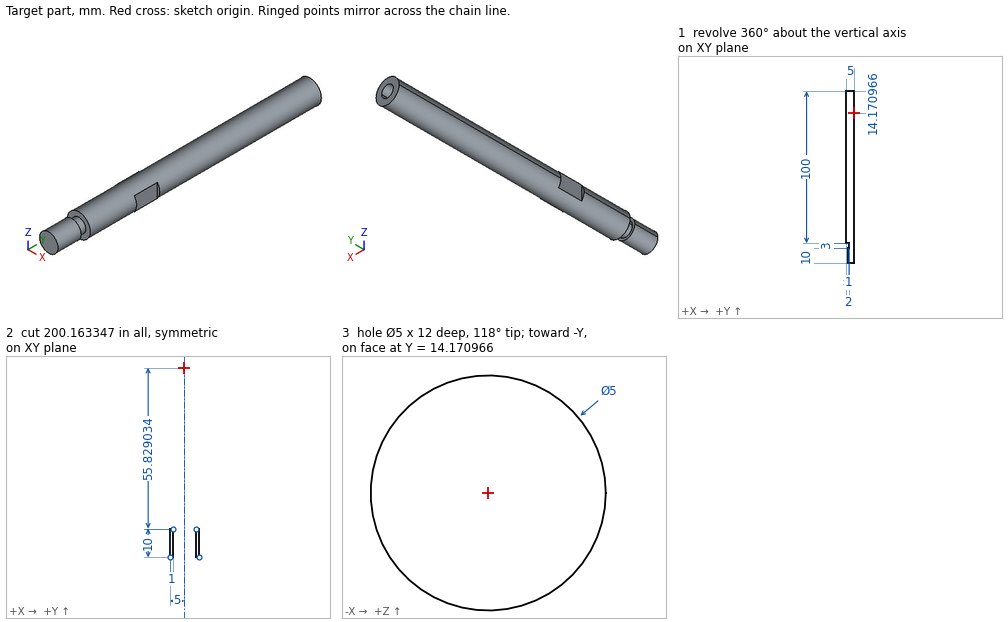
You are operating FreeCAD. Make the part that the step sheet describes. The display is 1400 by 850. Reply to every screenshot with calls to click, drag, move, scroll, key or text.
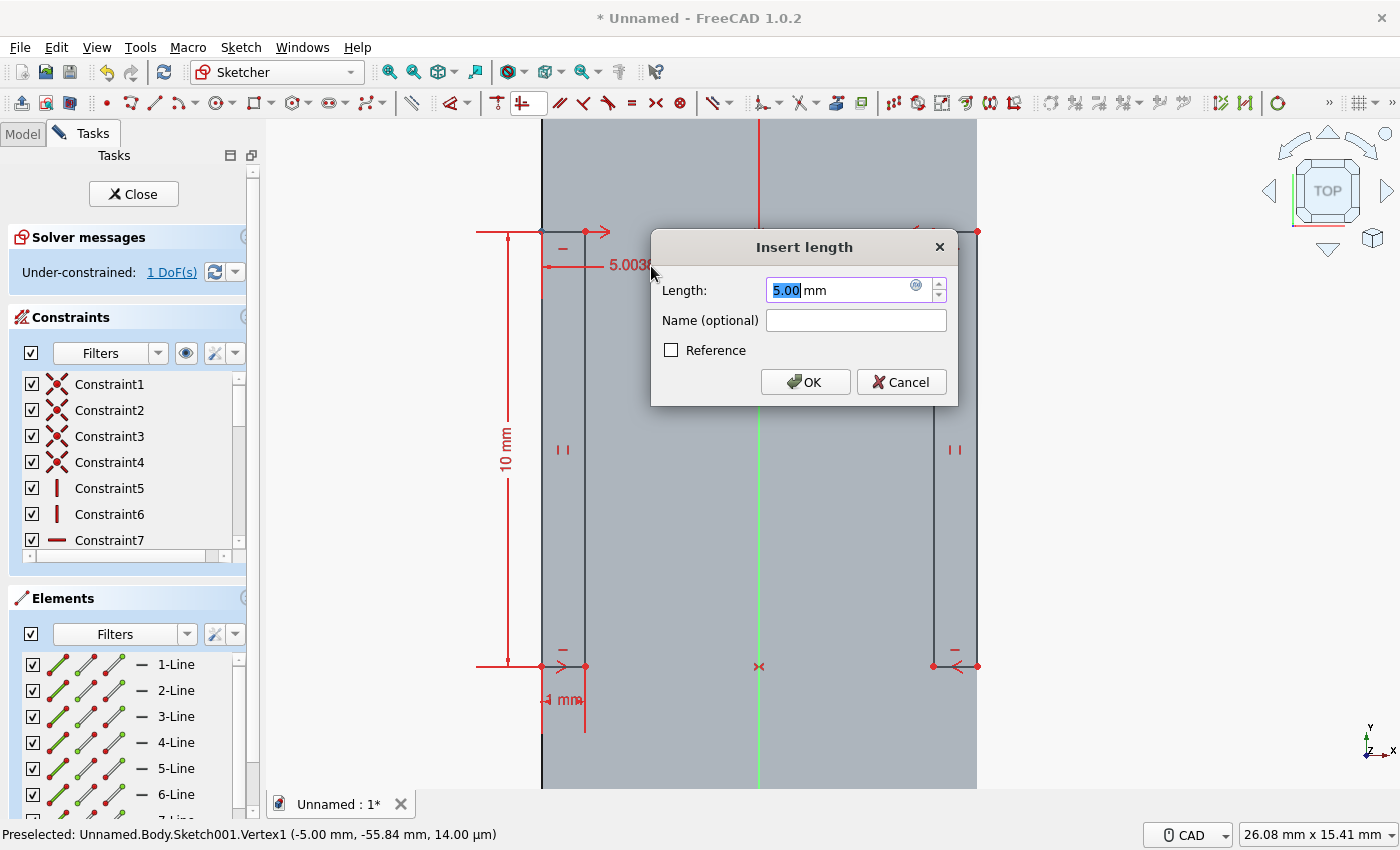
text(5)
key(Return)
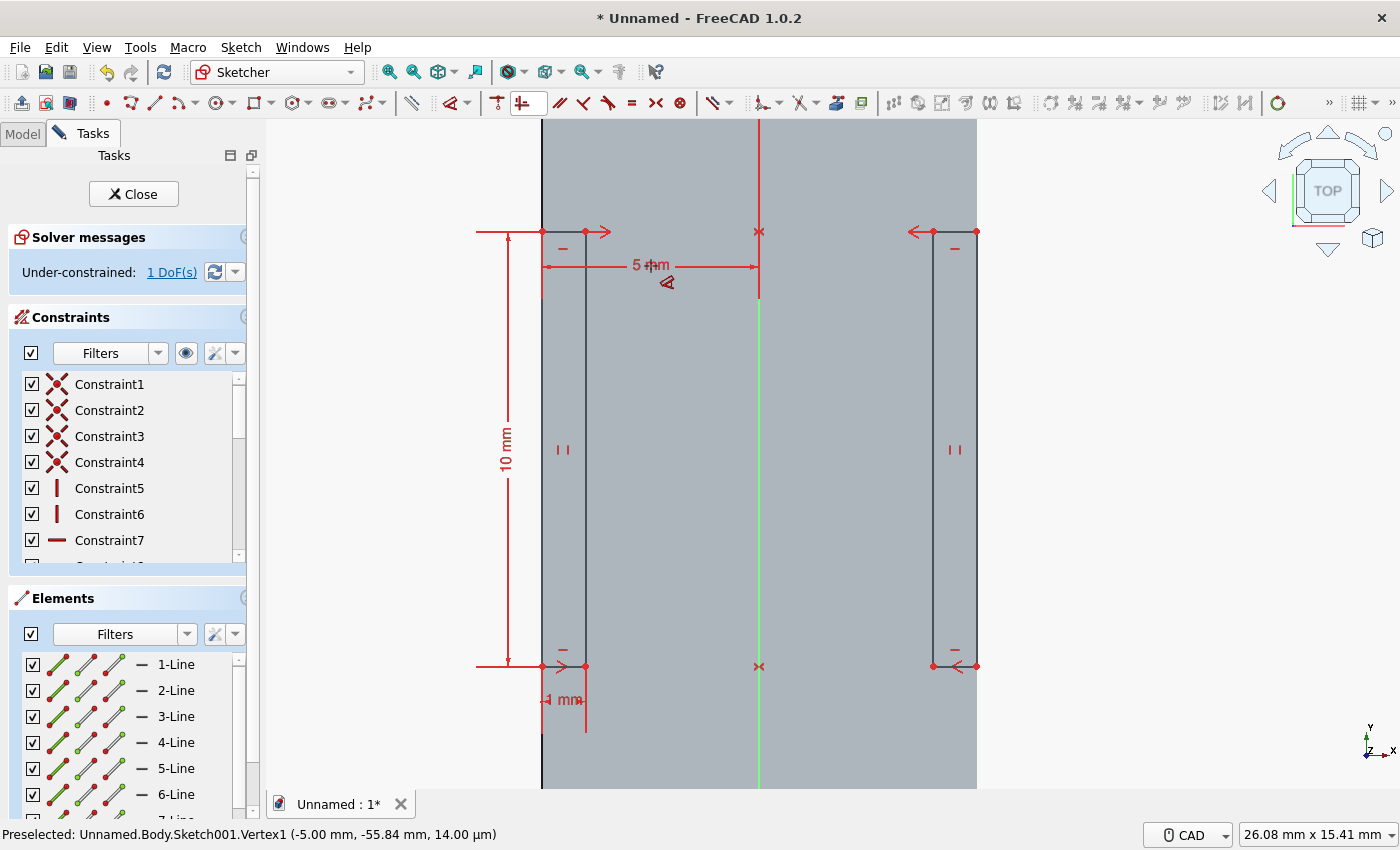
click(542, 232)
click(508, 189)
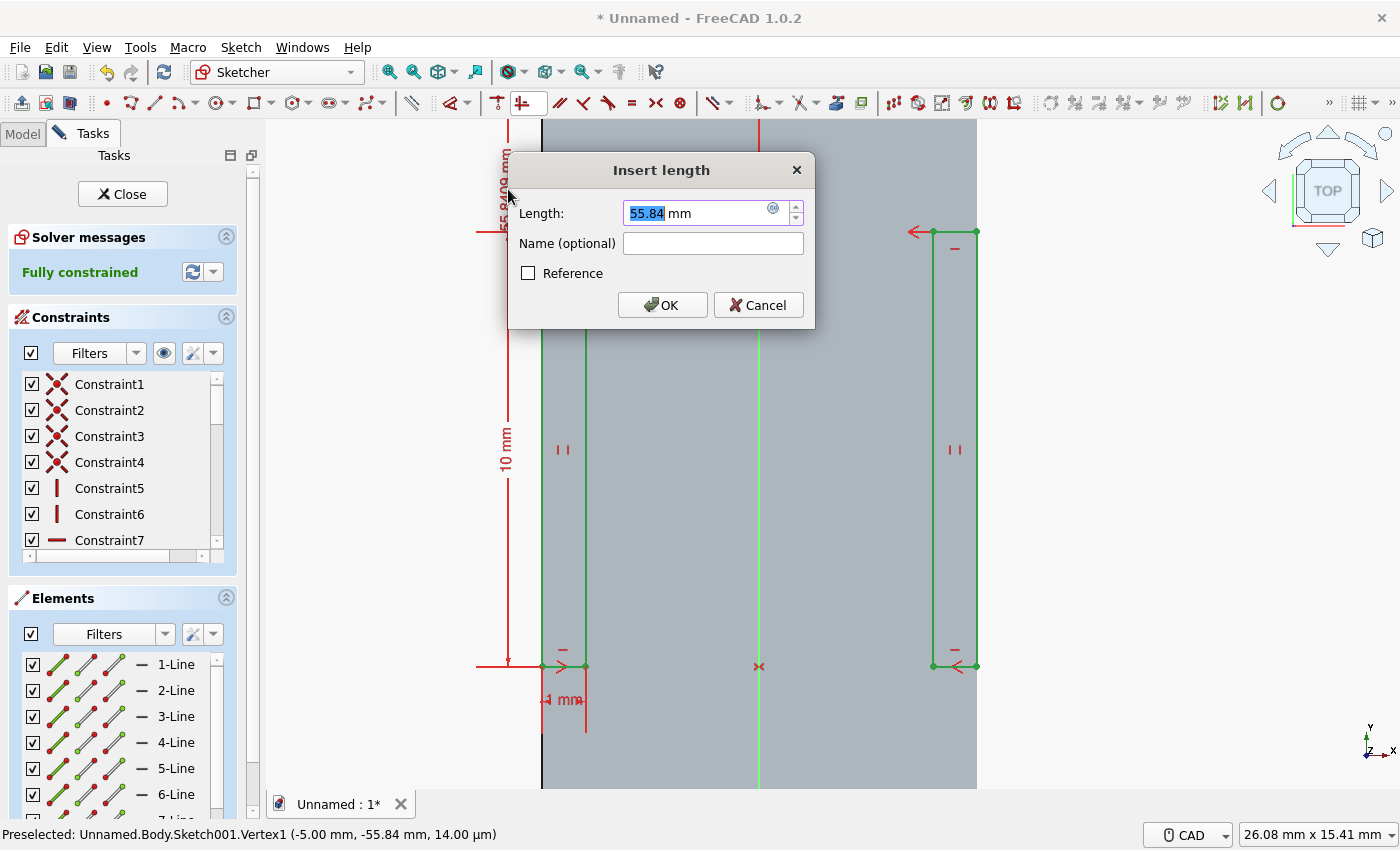
text(55.829034)
key(Return)
key(Escape)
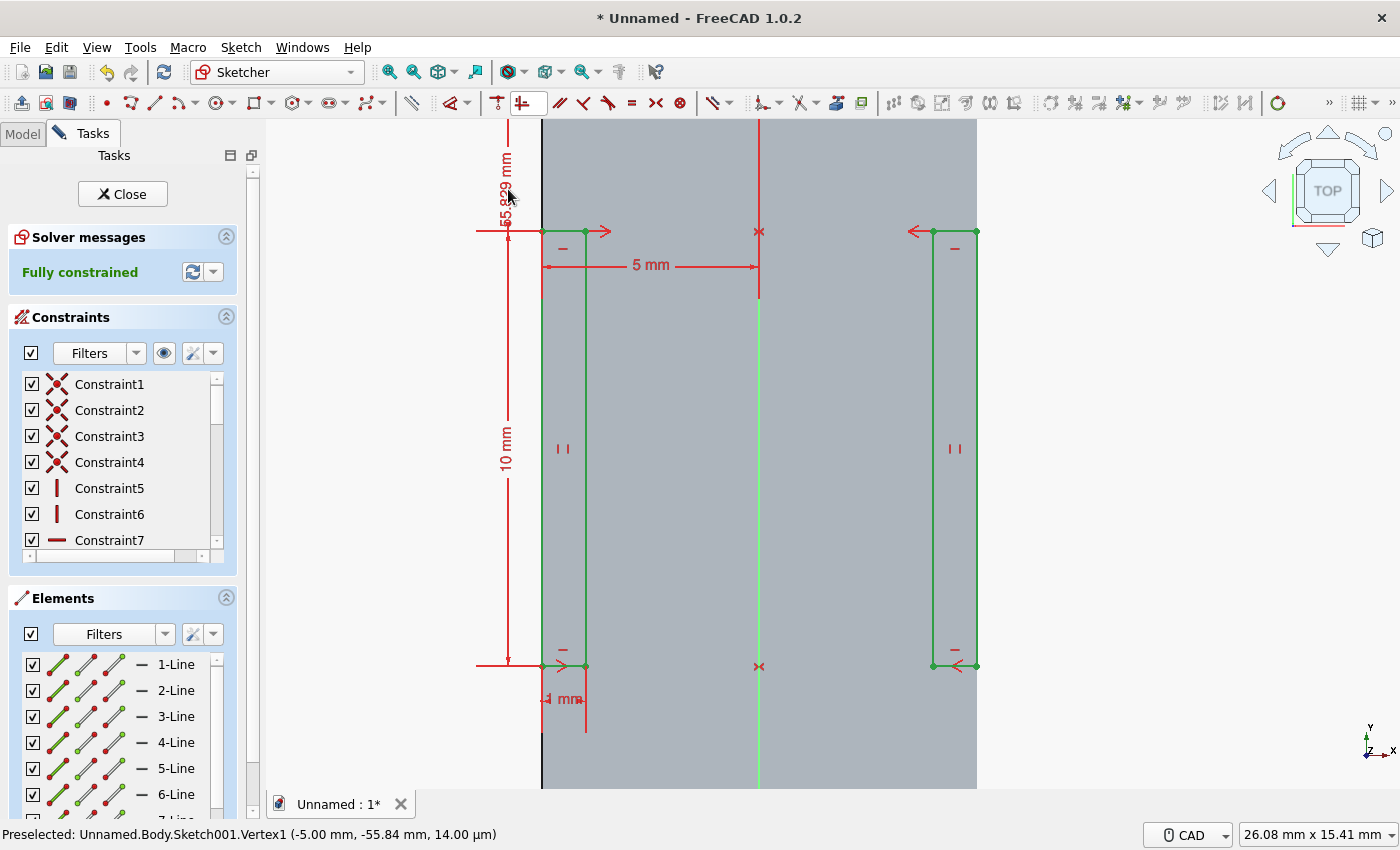
click(123, 194)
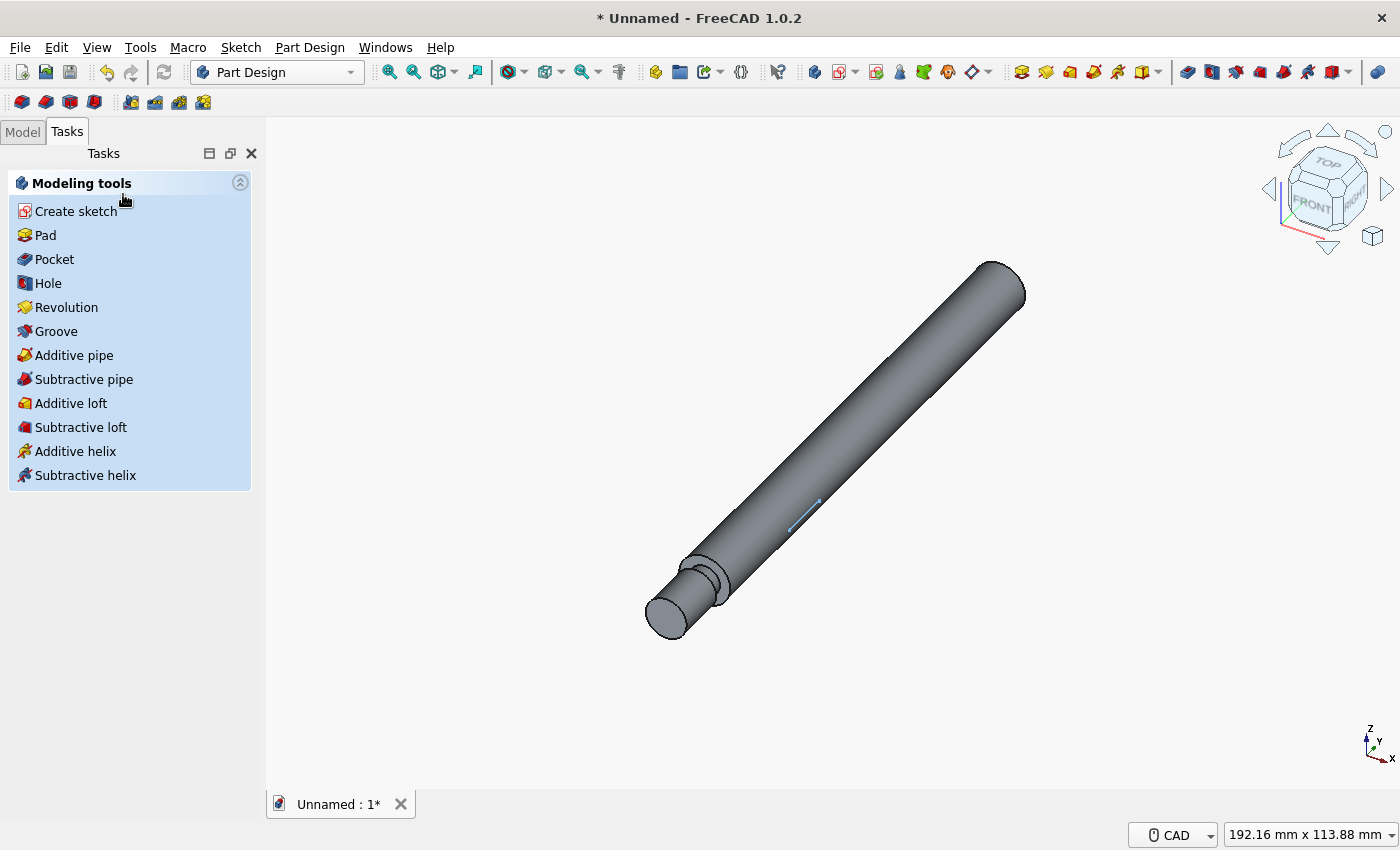
click(1188, 72)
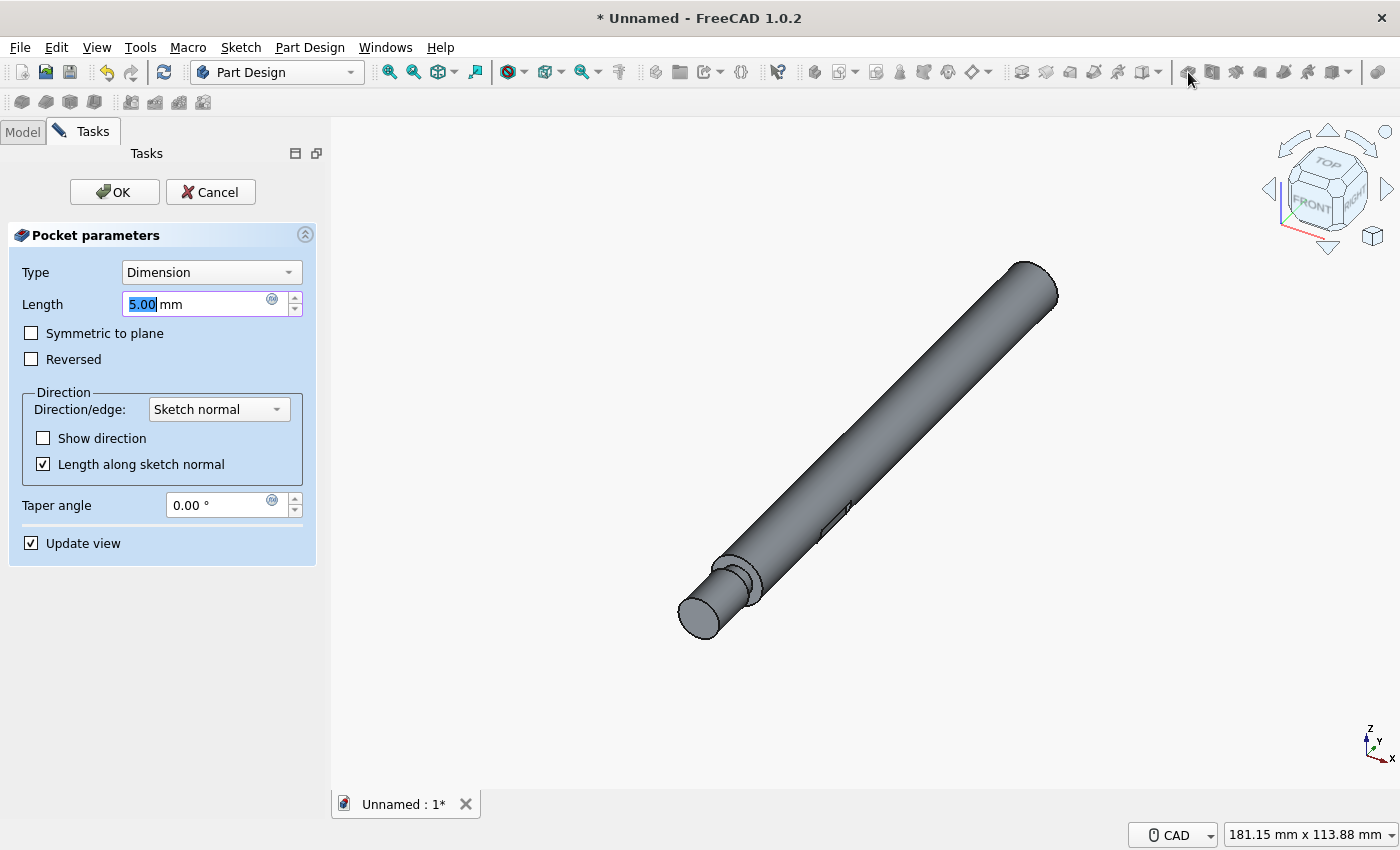
text(200.163347)
key(Tab)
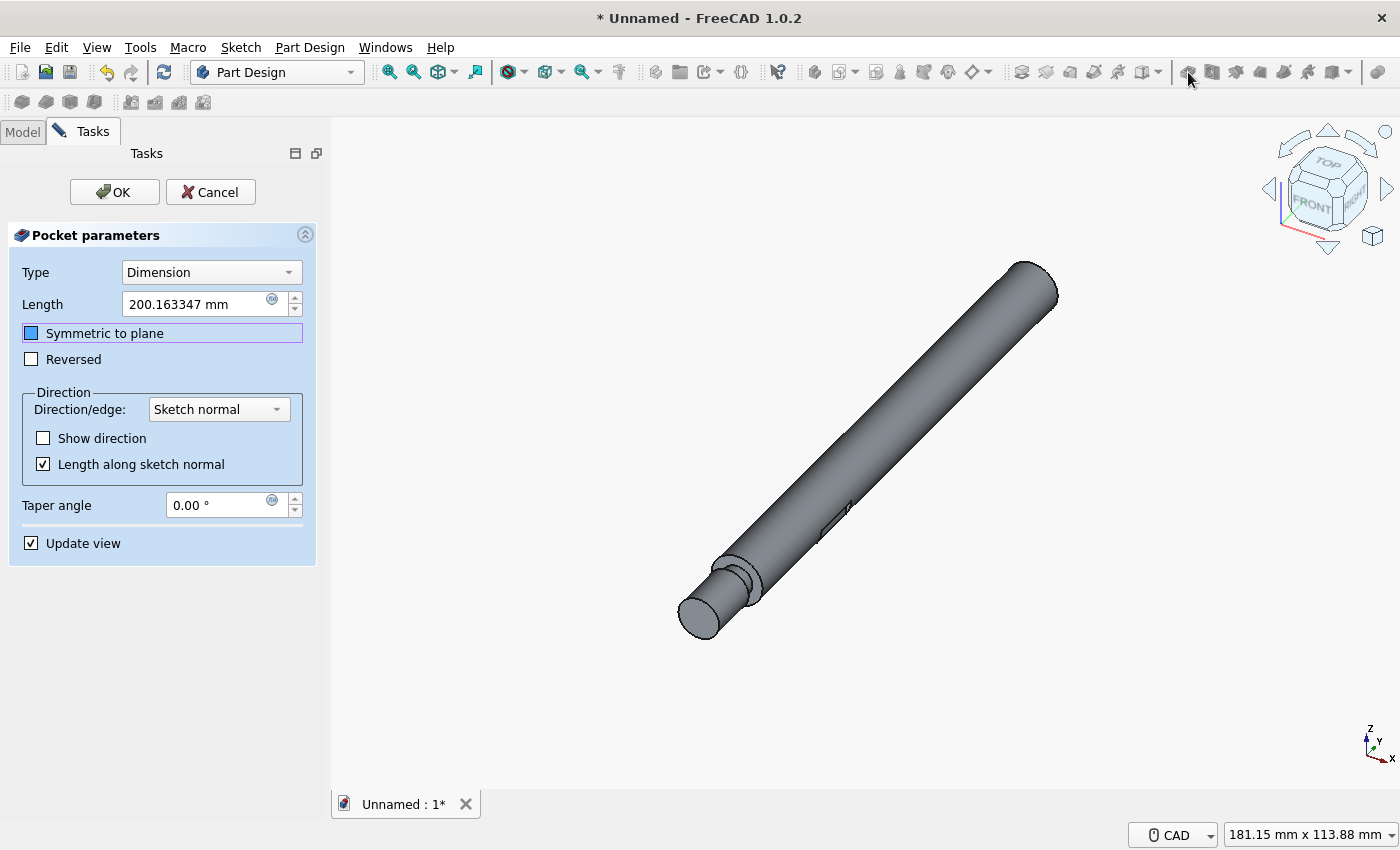
click(30, 333)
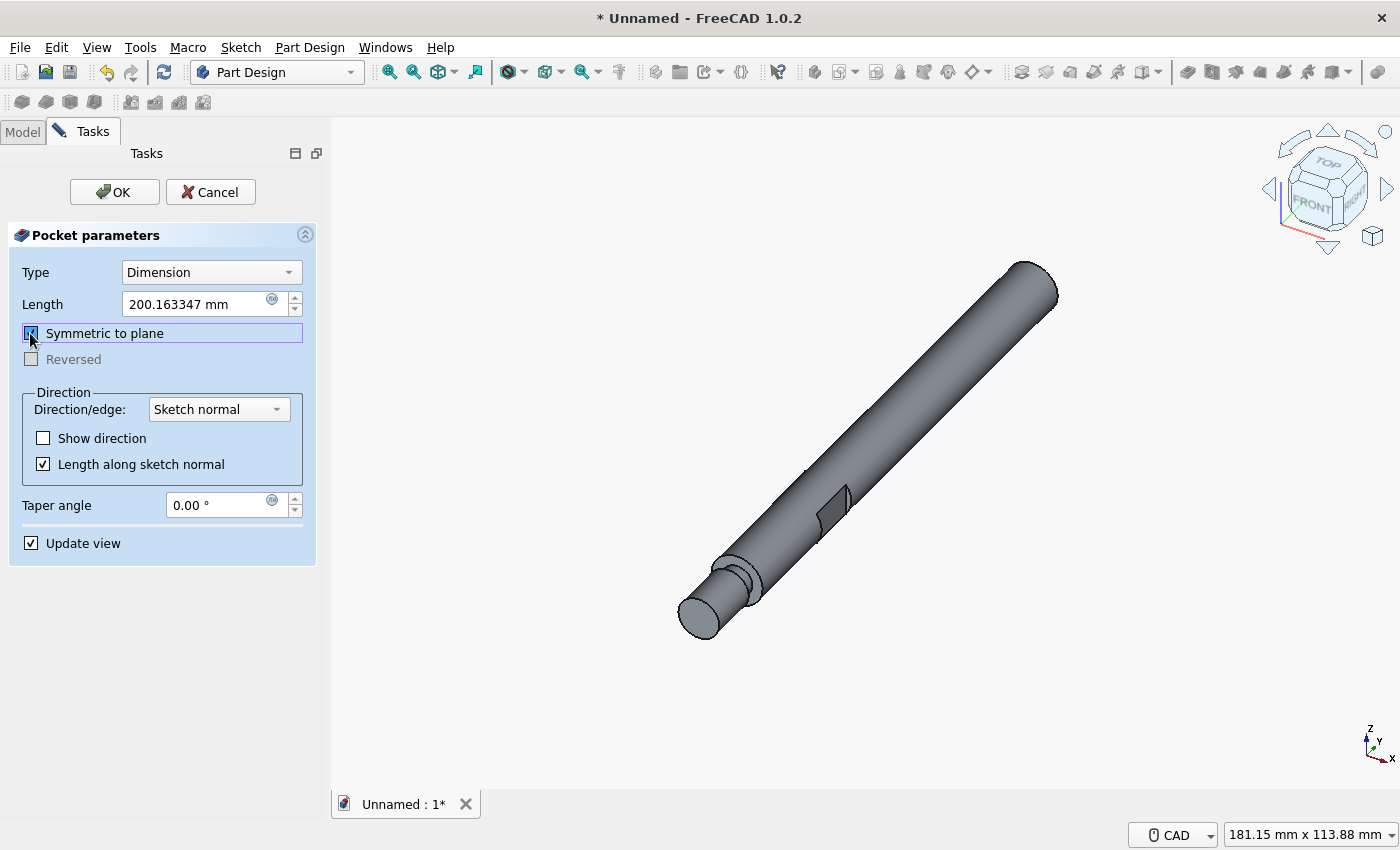
click(115, 192)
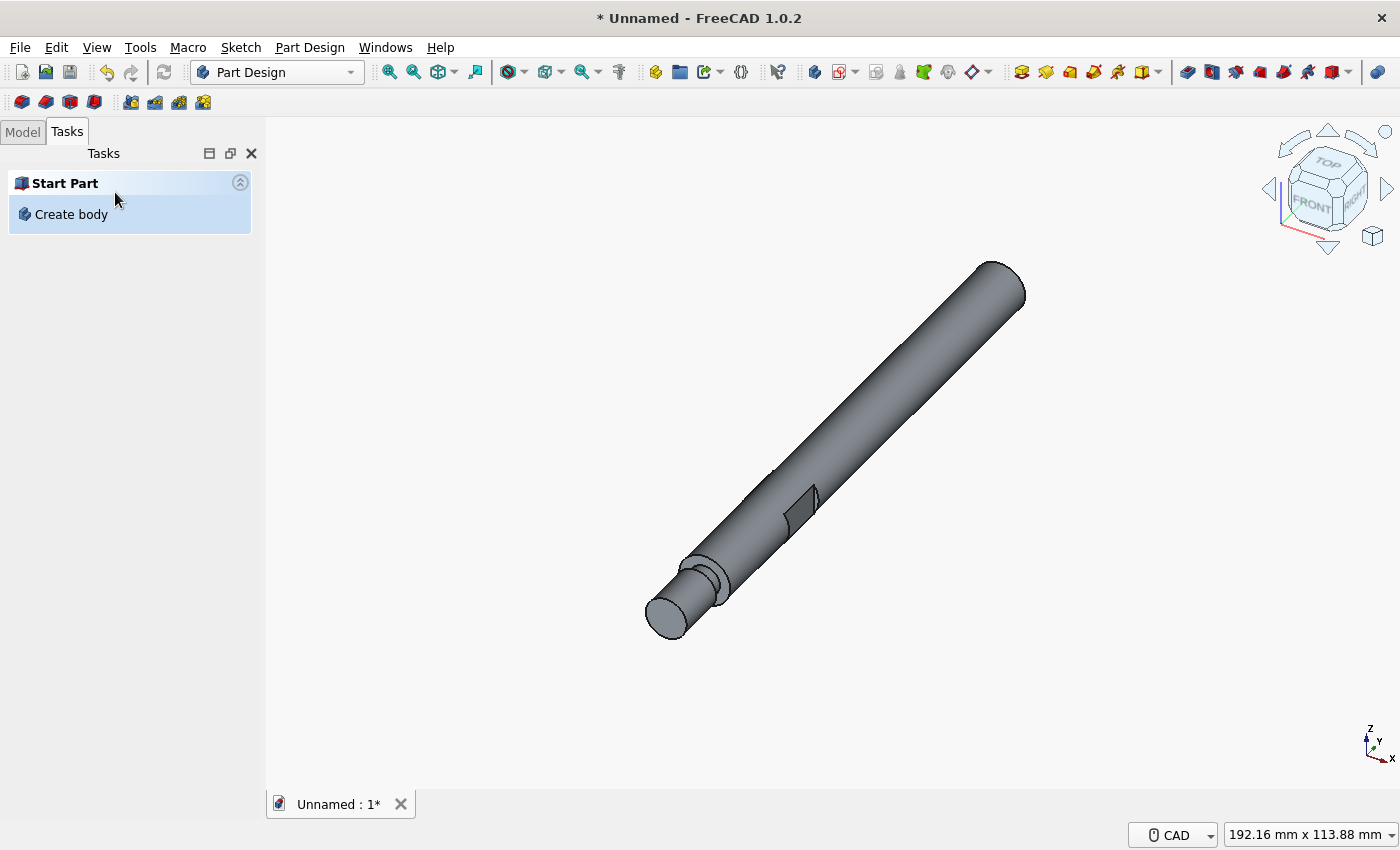
key(4)